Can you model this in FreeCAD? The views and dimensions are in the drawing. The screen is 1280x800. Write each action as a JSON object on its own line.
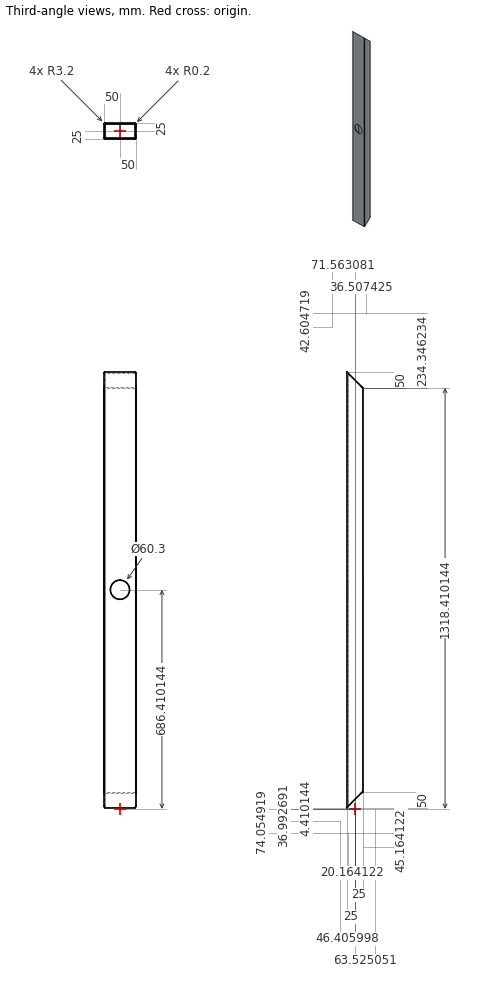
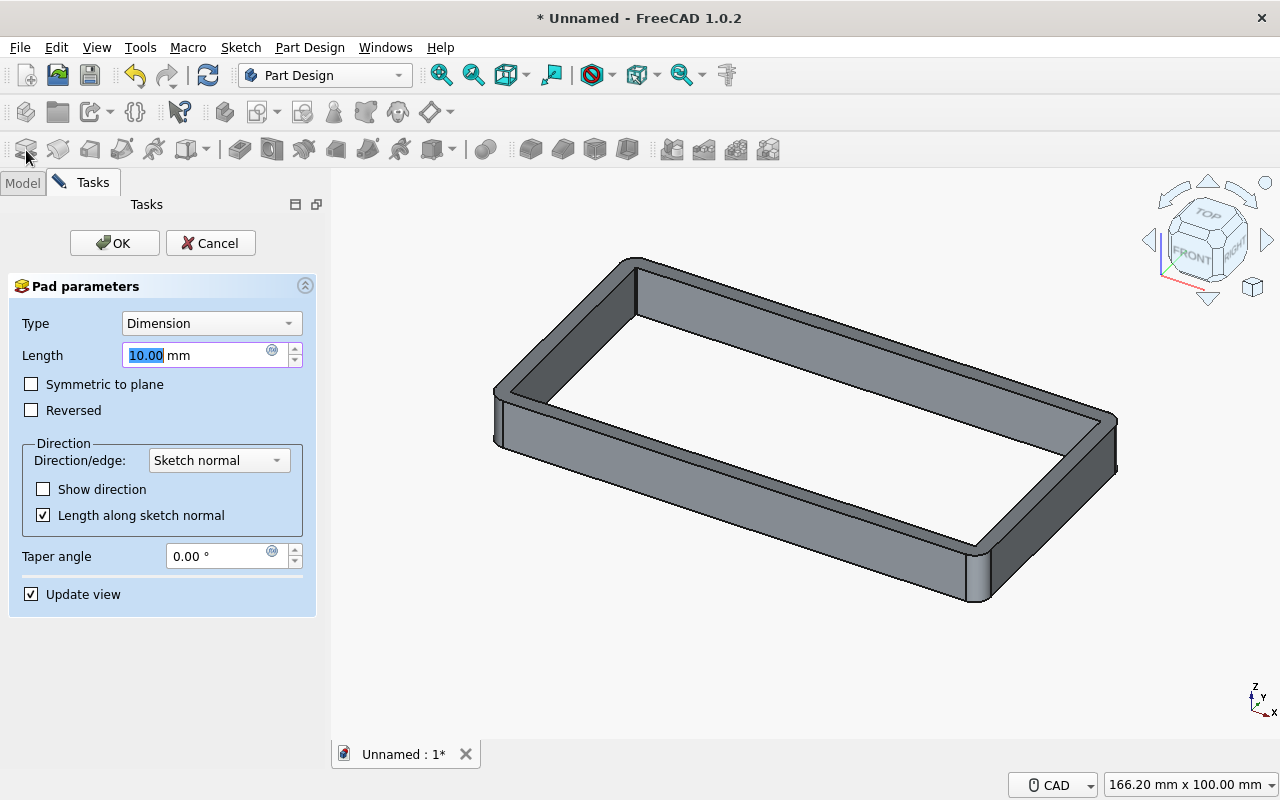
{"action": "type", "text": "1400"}
{"action": "key", "text": "Tab"}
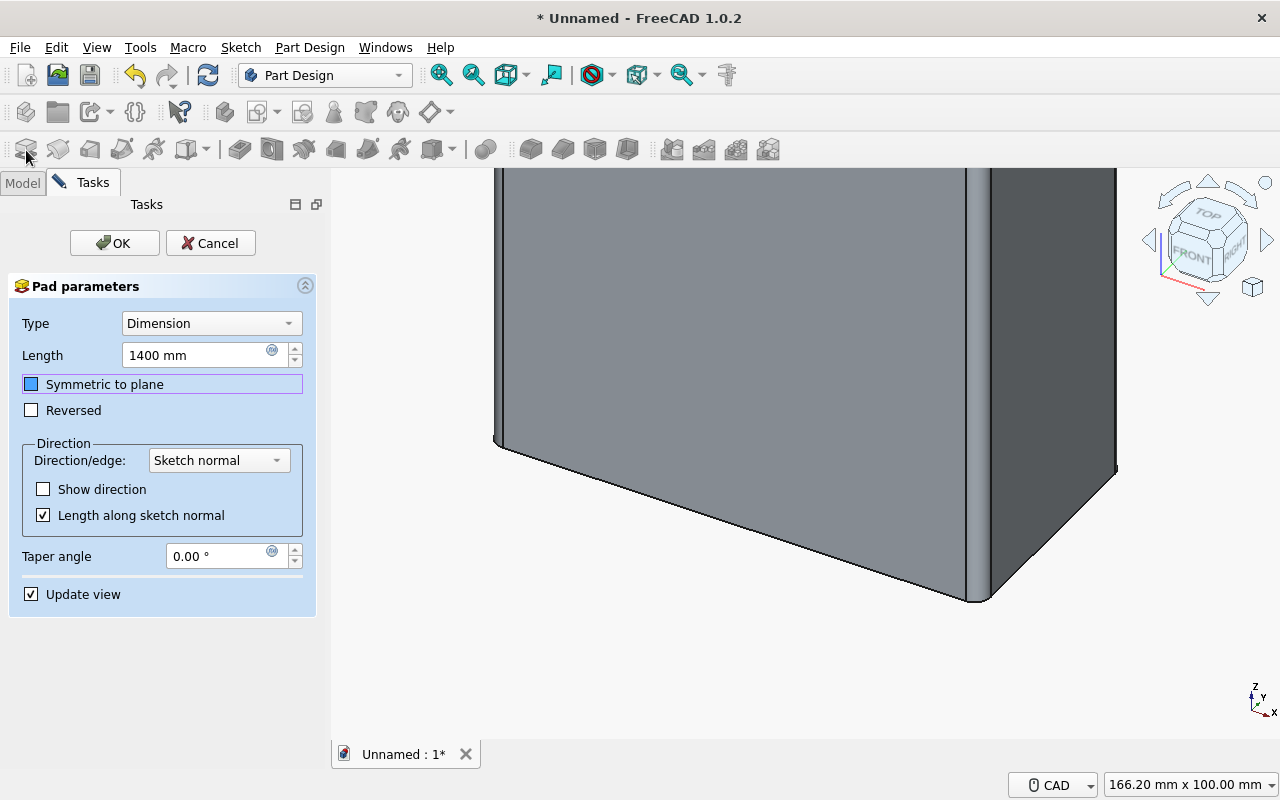
{"action": "left_click", "coordinate": [115, 243]}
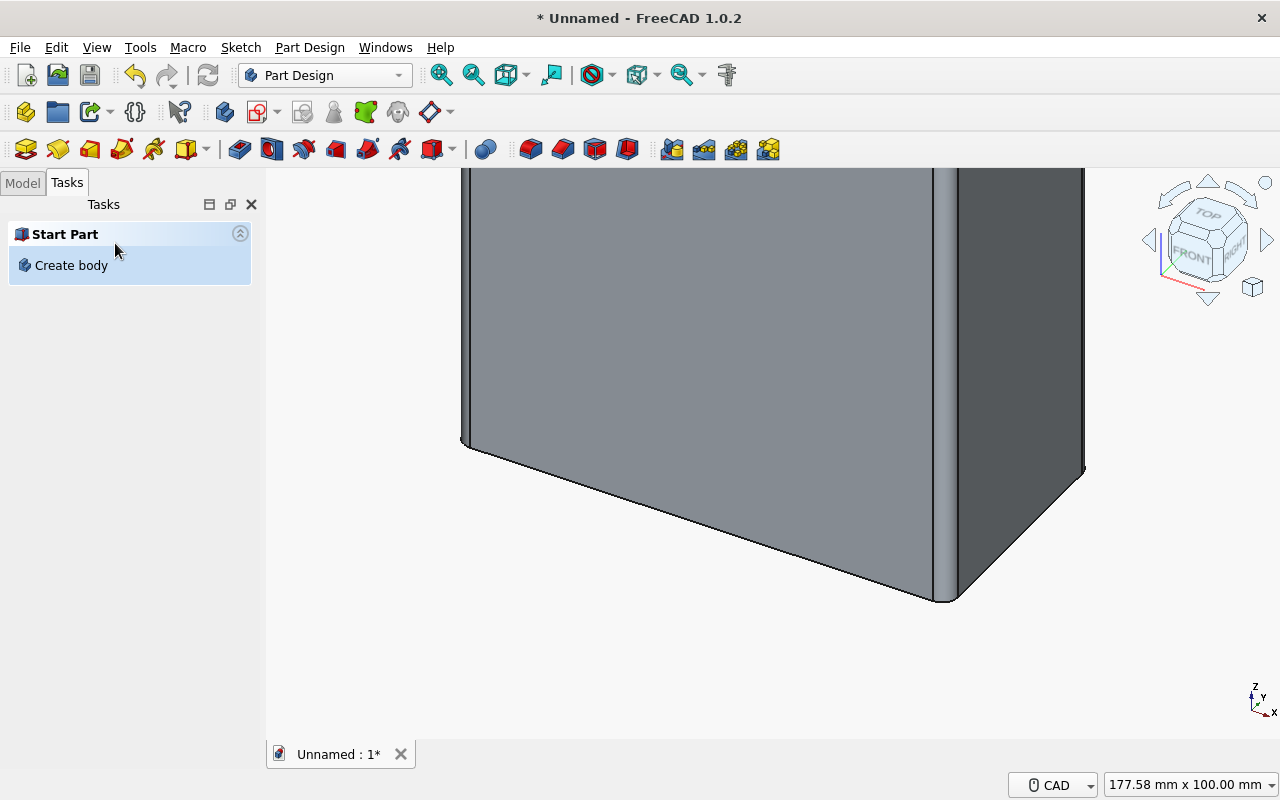
{"action": "left_click", "coordinate": [442, 76]}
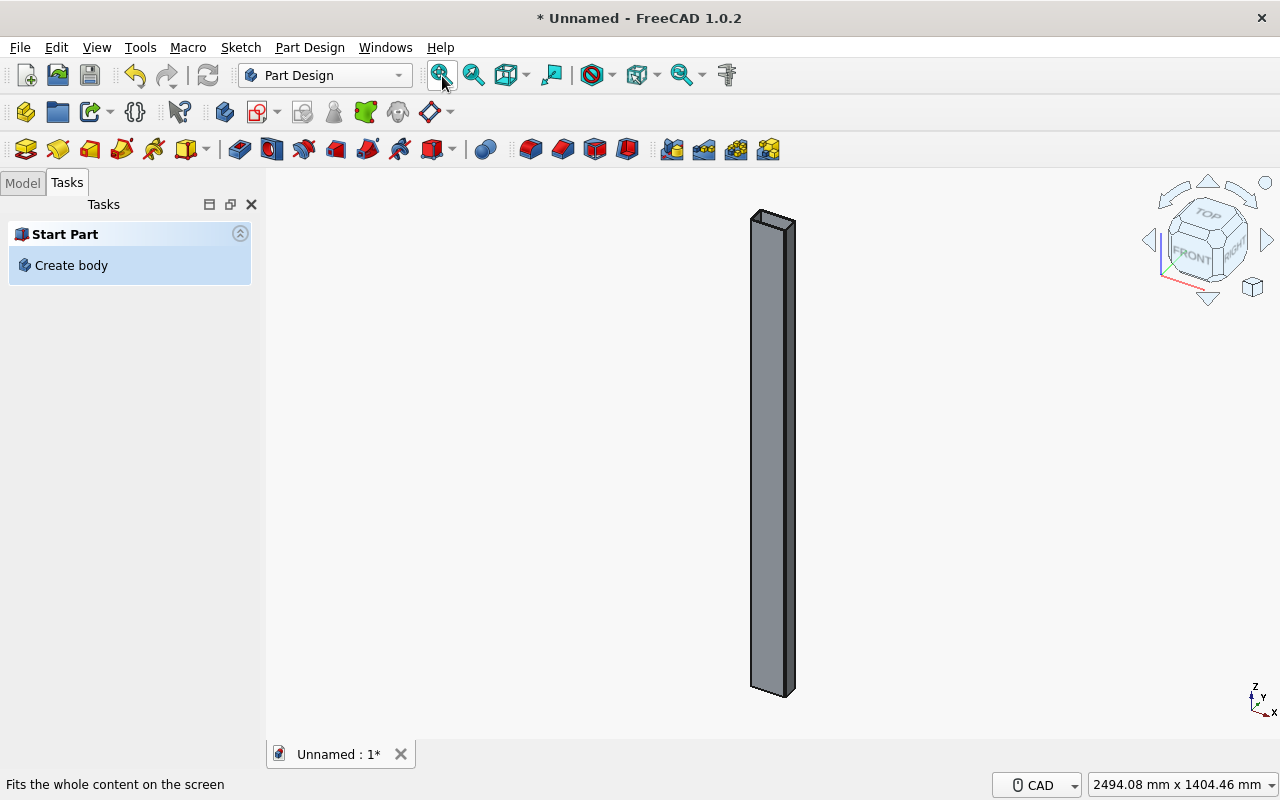
{"action": "key", "text": "0"}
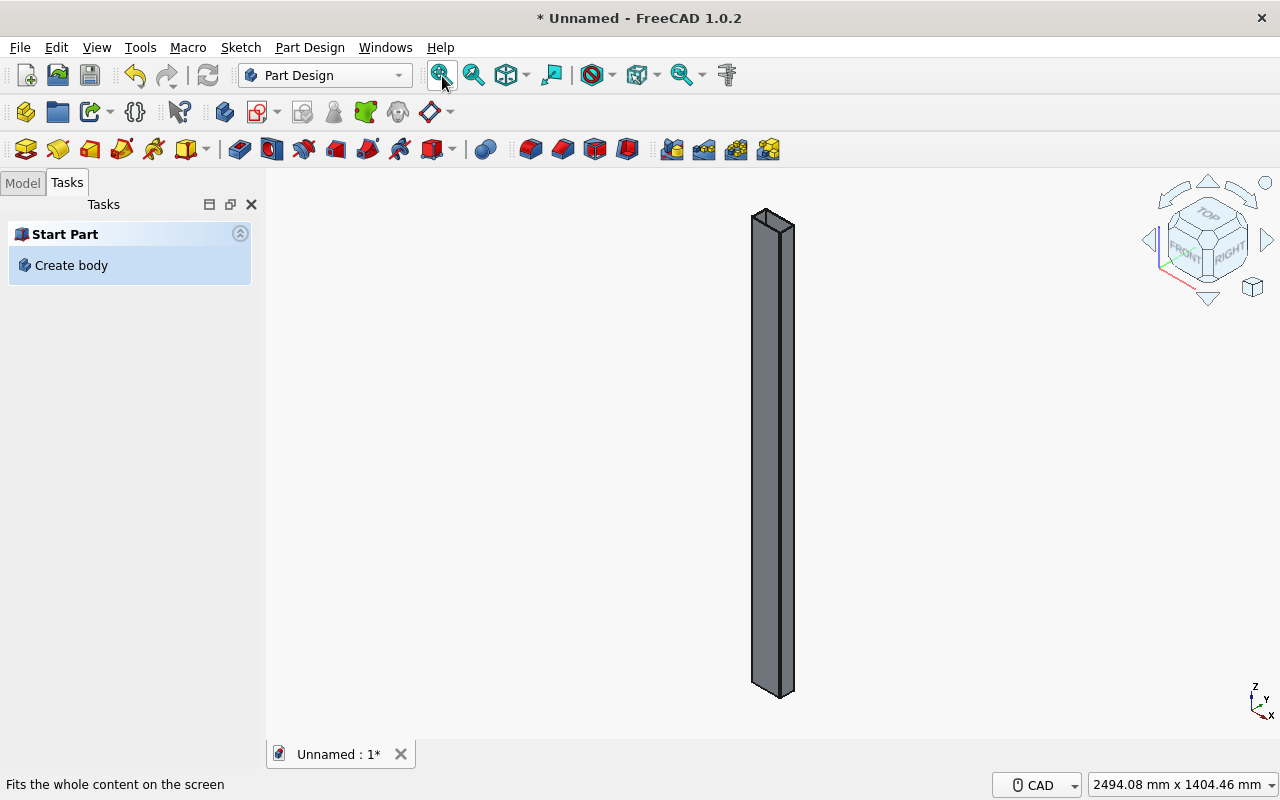
{"action": "key", "text": "3"}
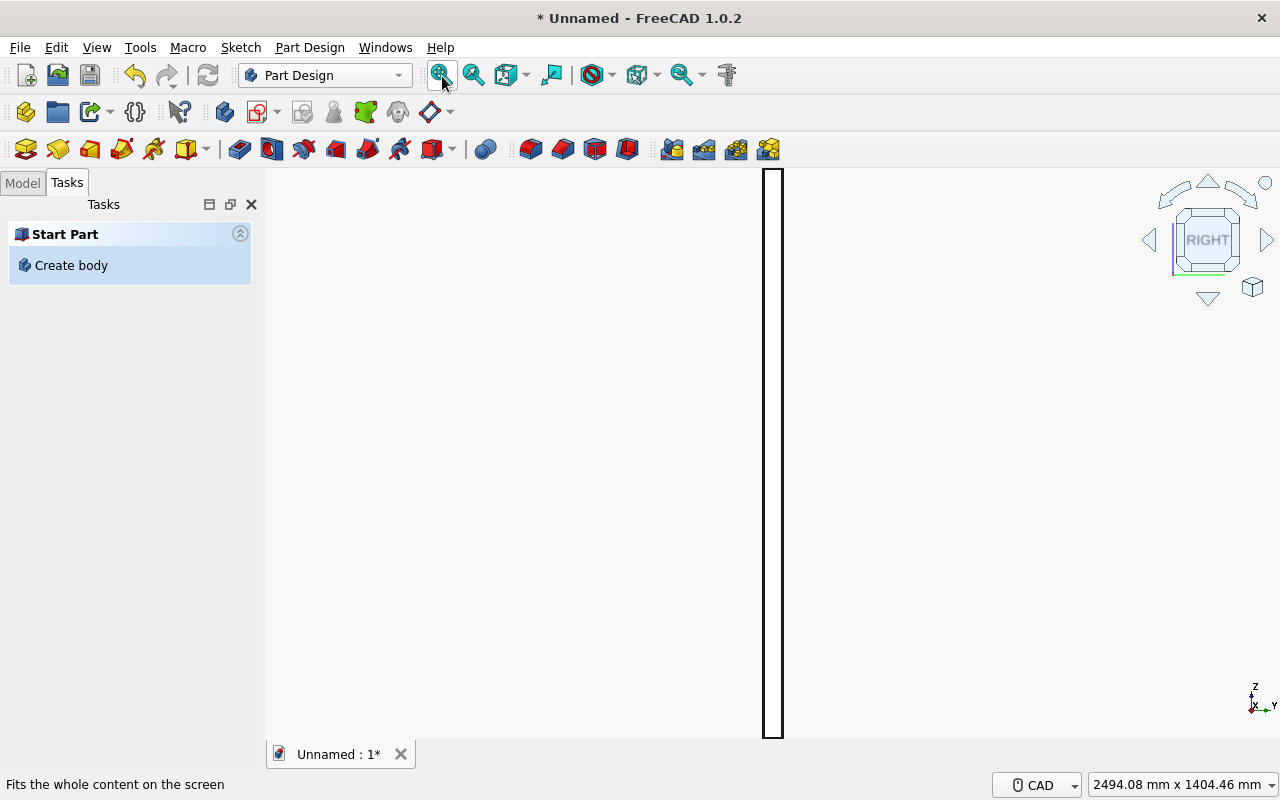
{"action": "left_click", "coordinate": [773, 209]}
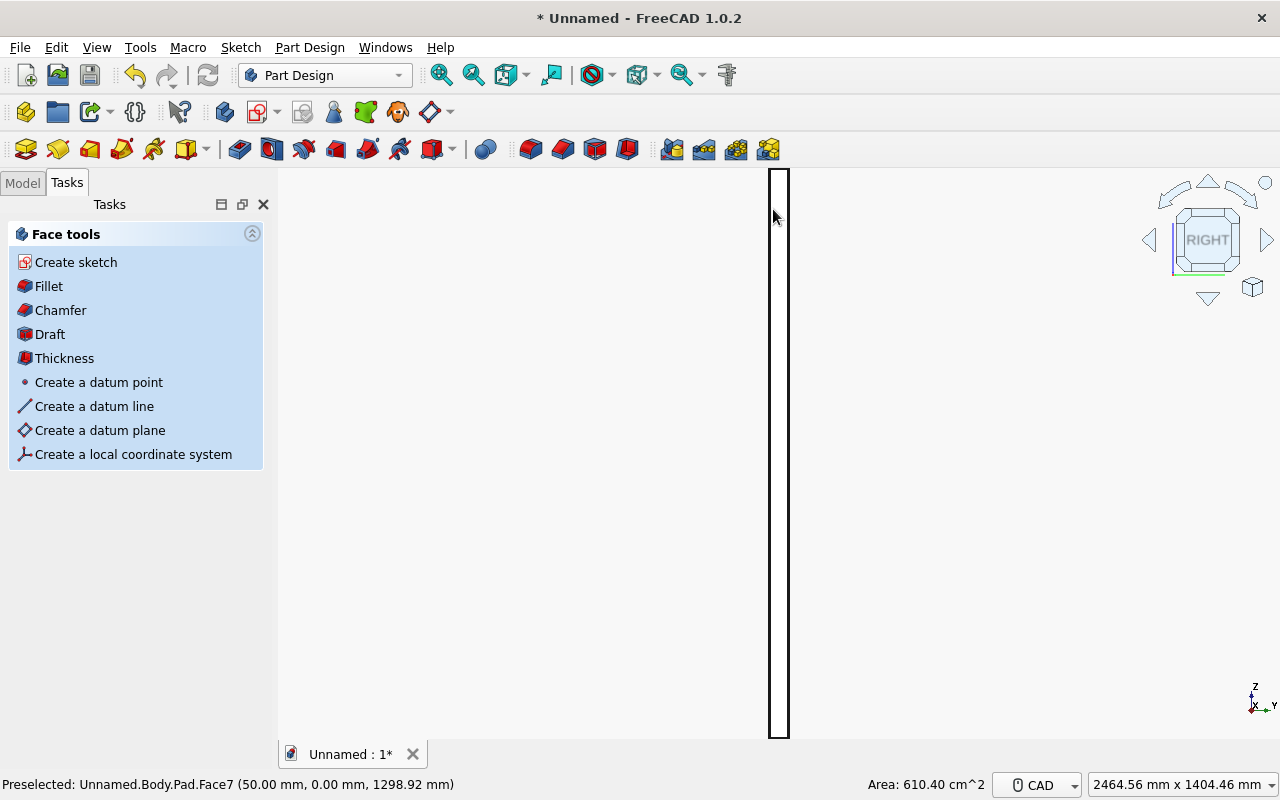
{"action": "left_click", "coordinate": [258, 112]}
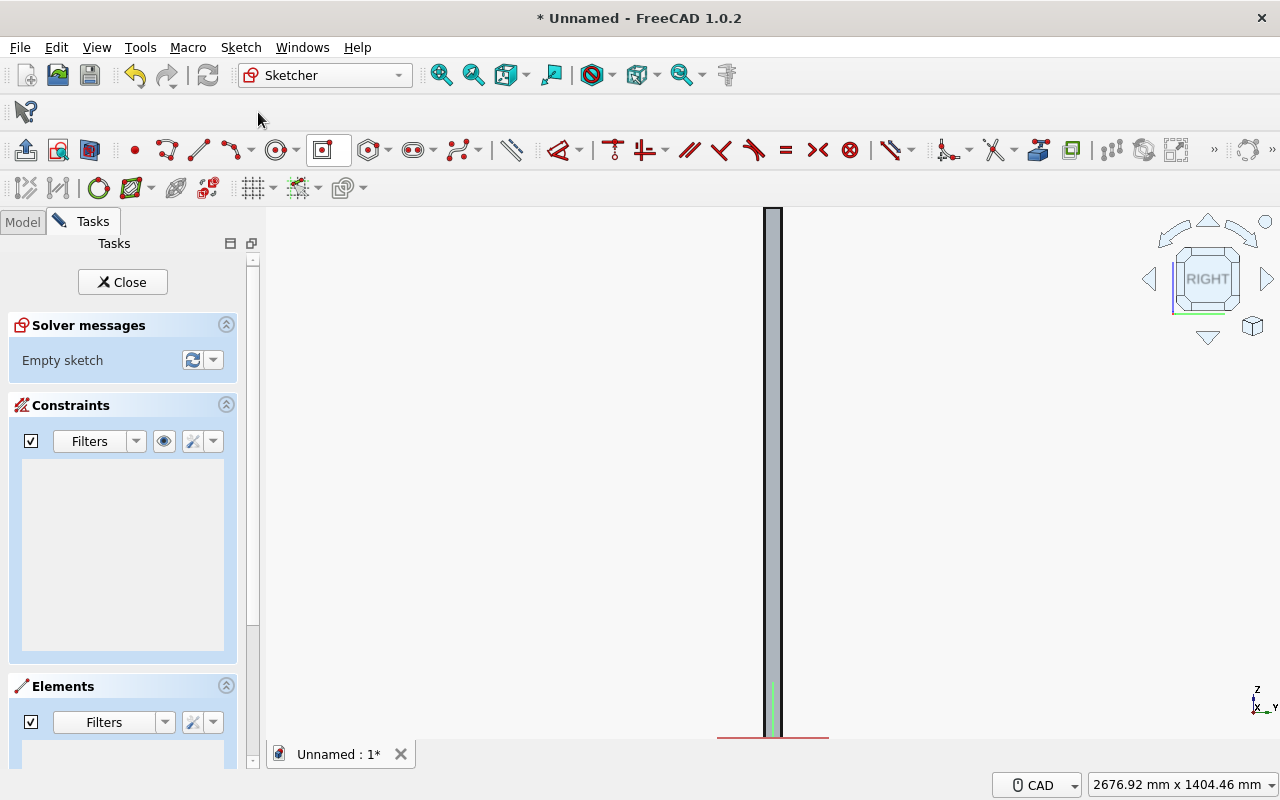
{"action": "scroll", "coordinate": [623, 481], "scroll_direction": "down", "scroll_amount": 3}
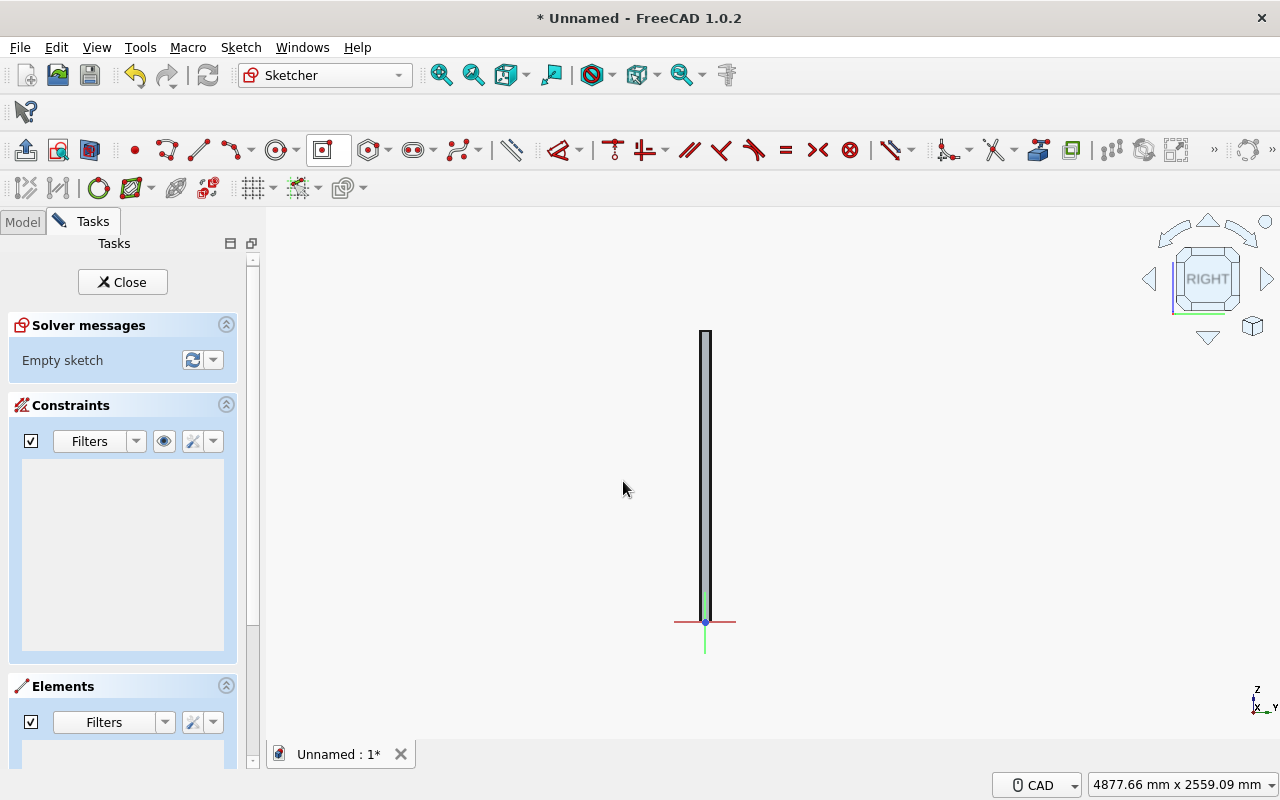
{"action": "left_click", "coordinate": [168, 150]}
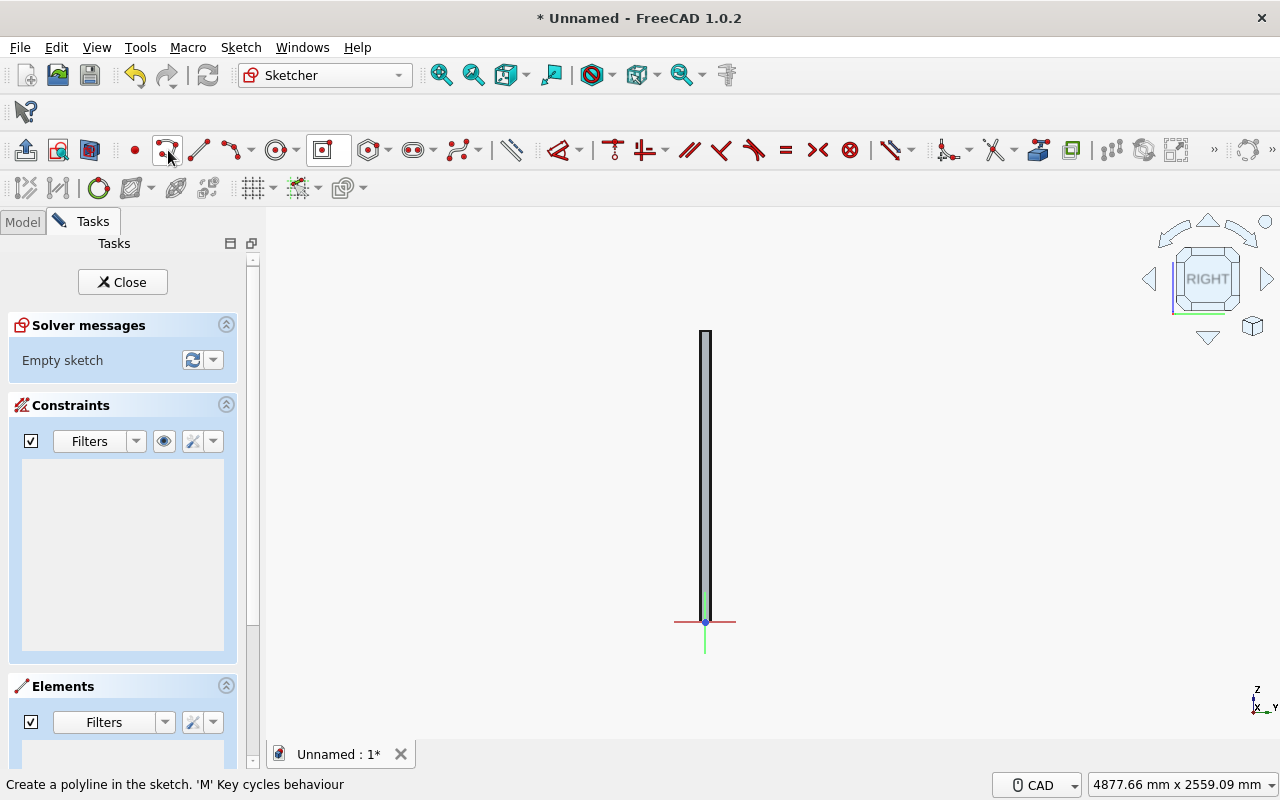
{"action": "scroll", "coordinate": [711, 348], "scroll_direction": "up", "scroll_amount": 6}